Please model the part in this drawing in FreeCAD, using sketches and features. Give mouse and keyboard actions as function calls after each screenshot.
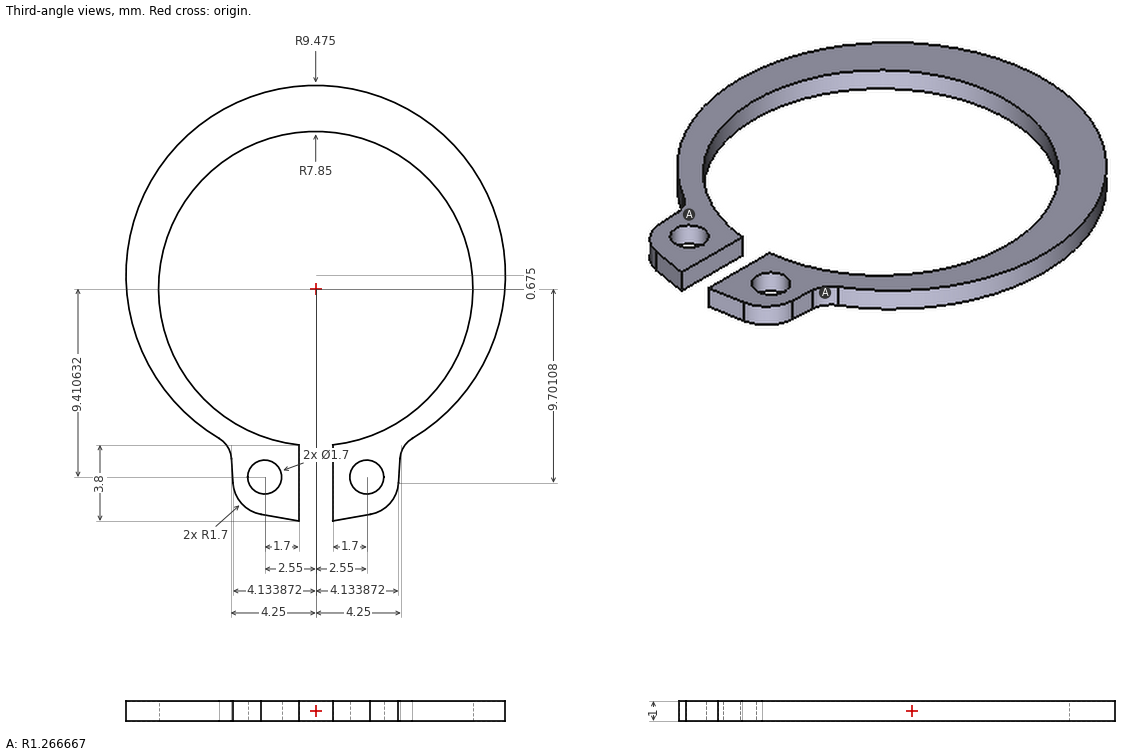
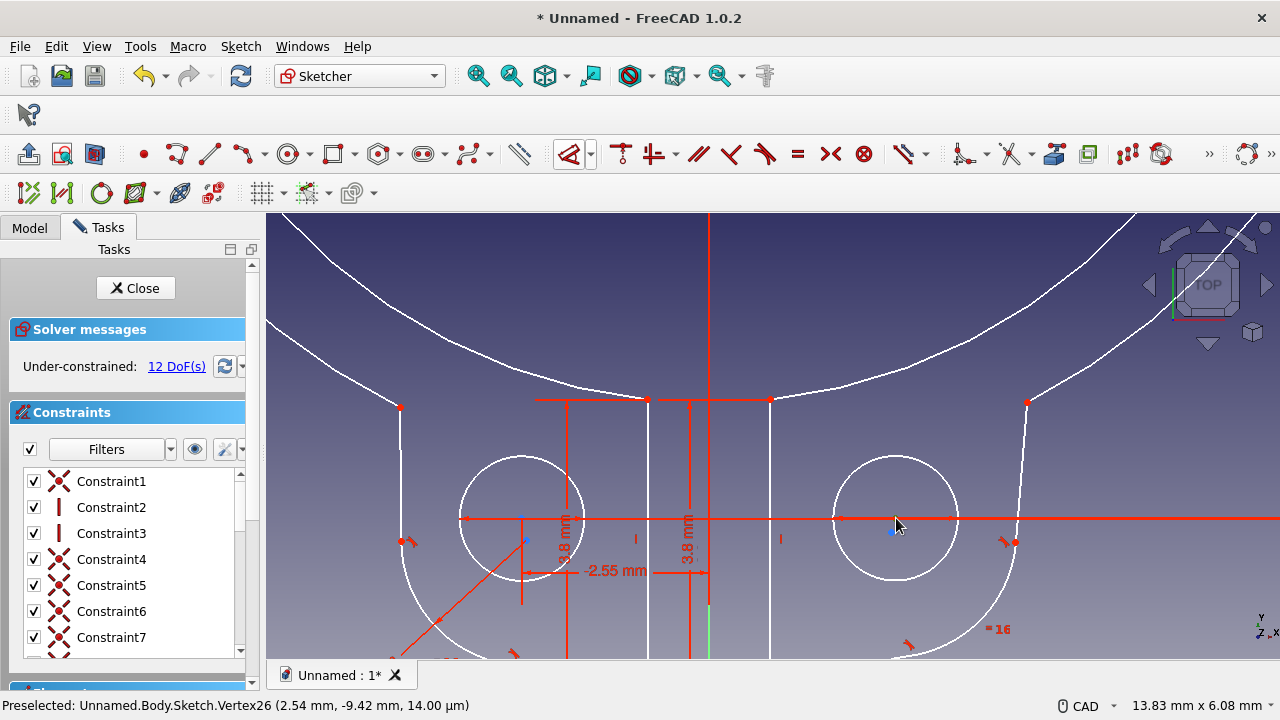
key(l)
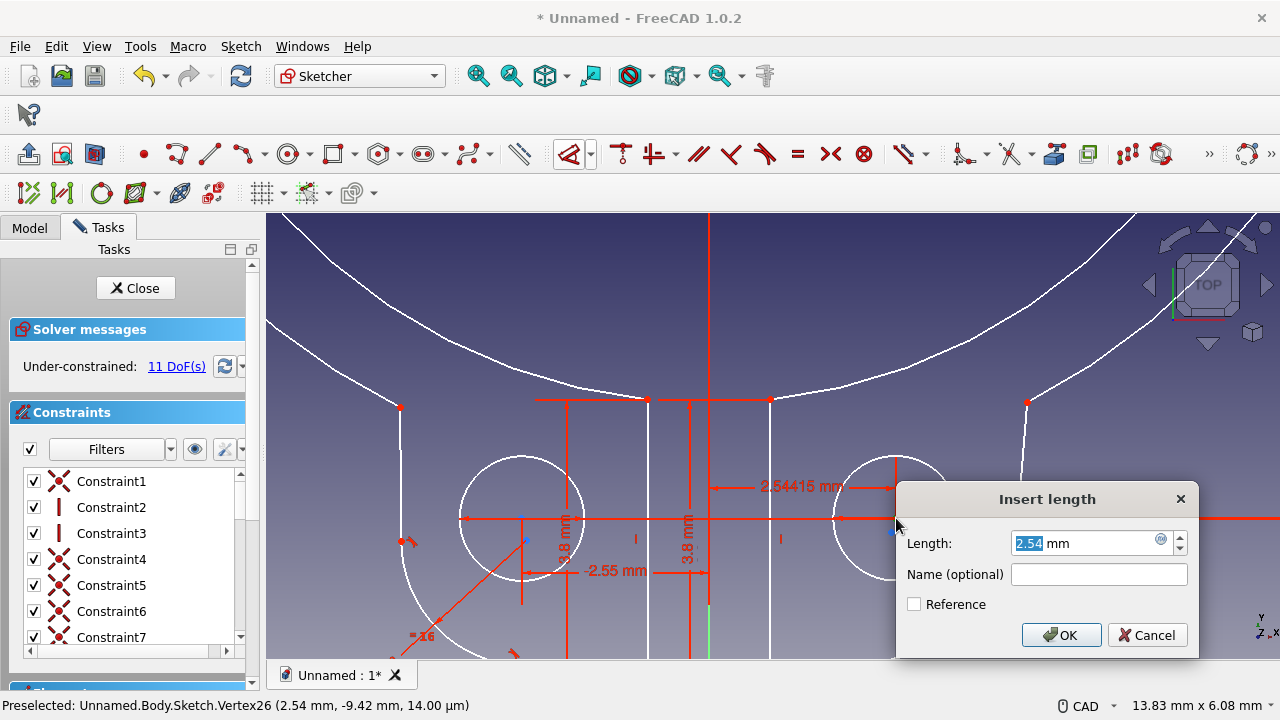
text(2.55)
key(Return)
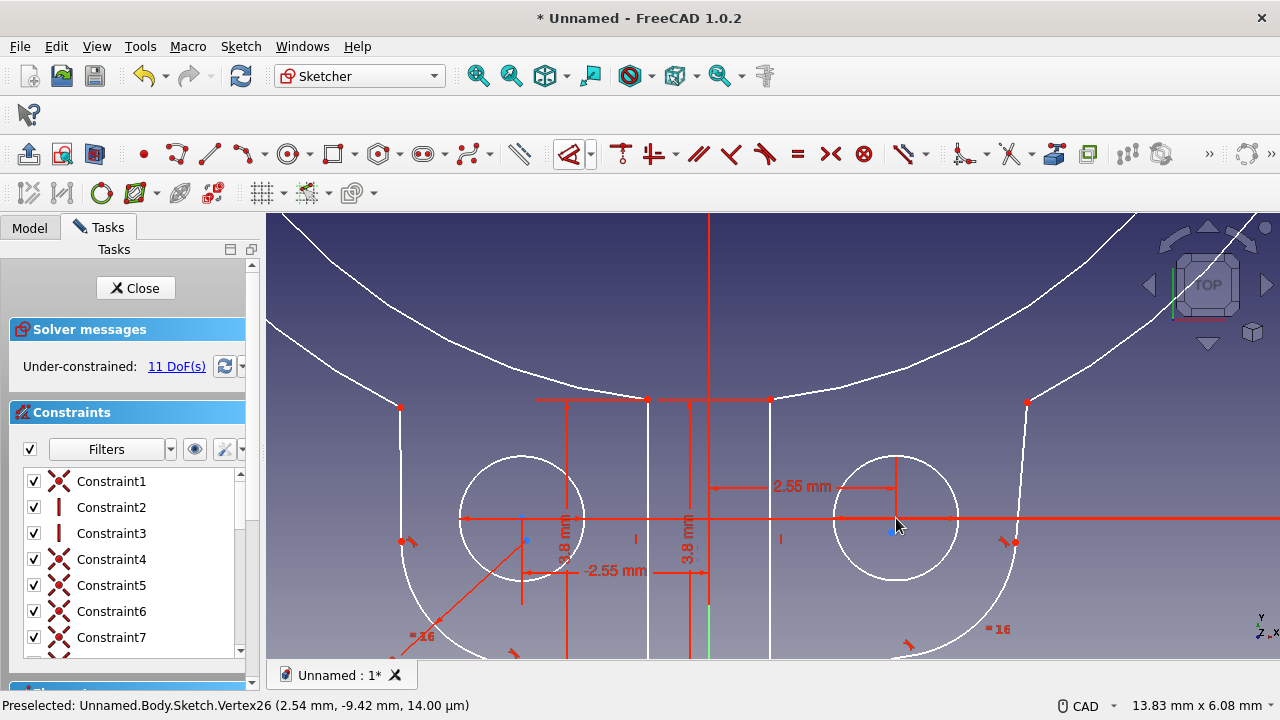
scroll(704, 546, down, 9)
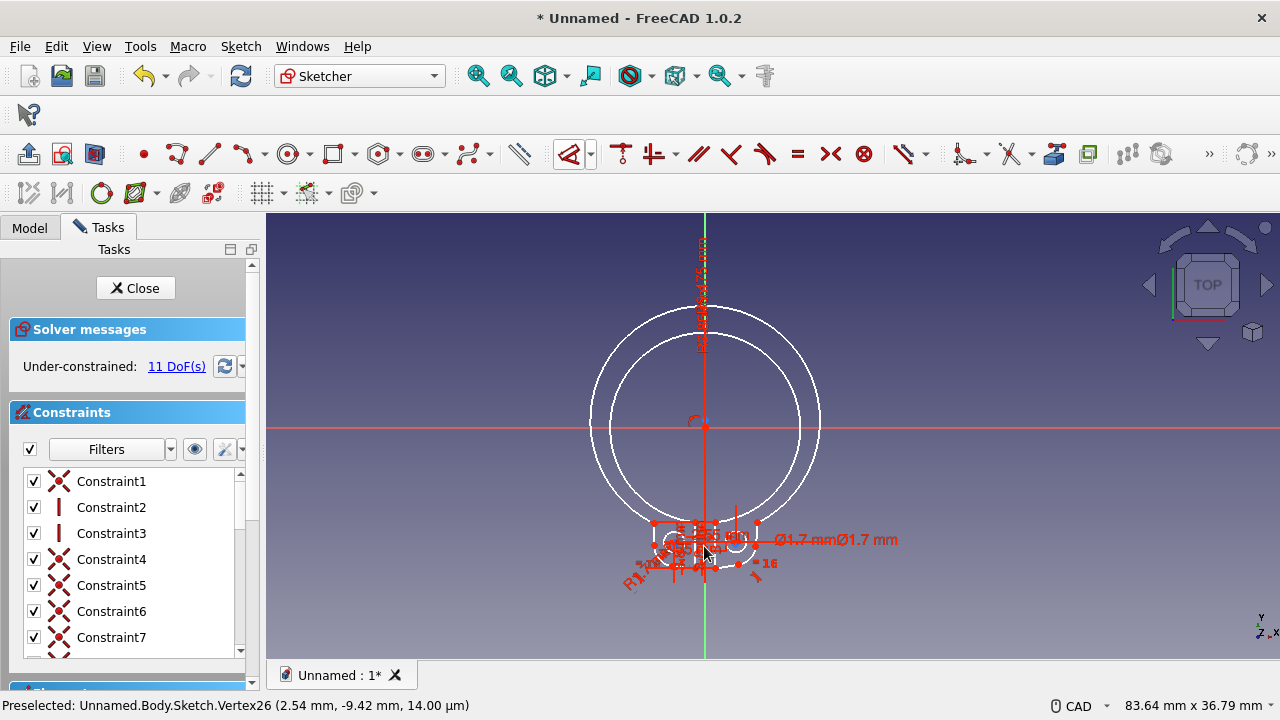
scroll(695, 522, up, 4)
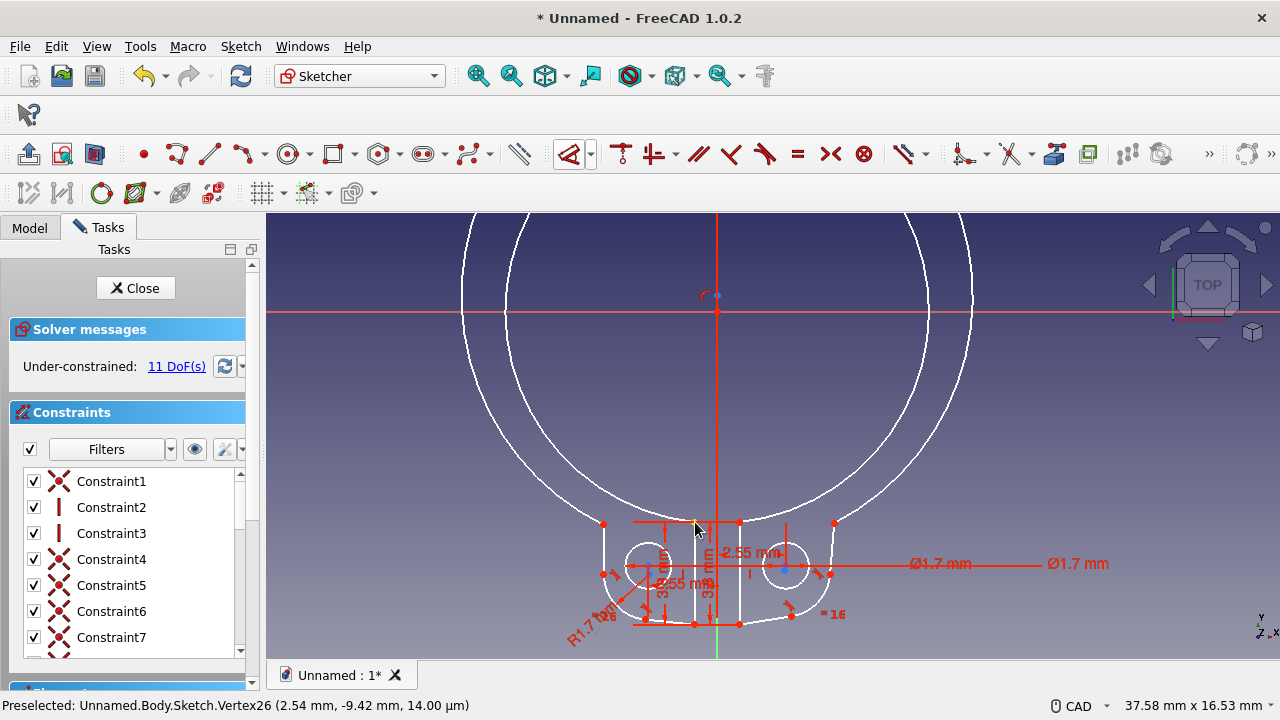
click(695, 522)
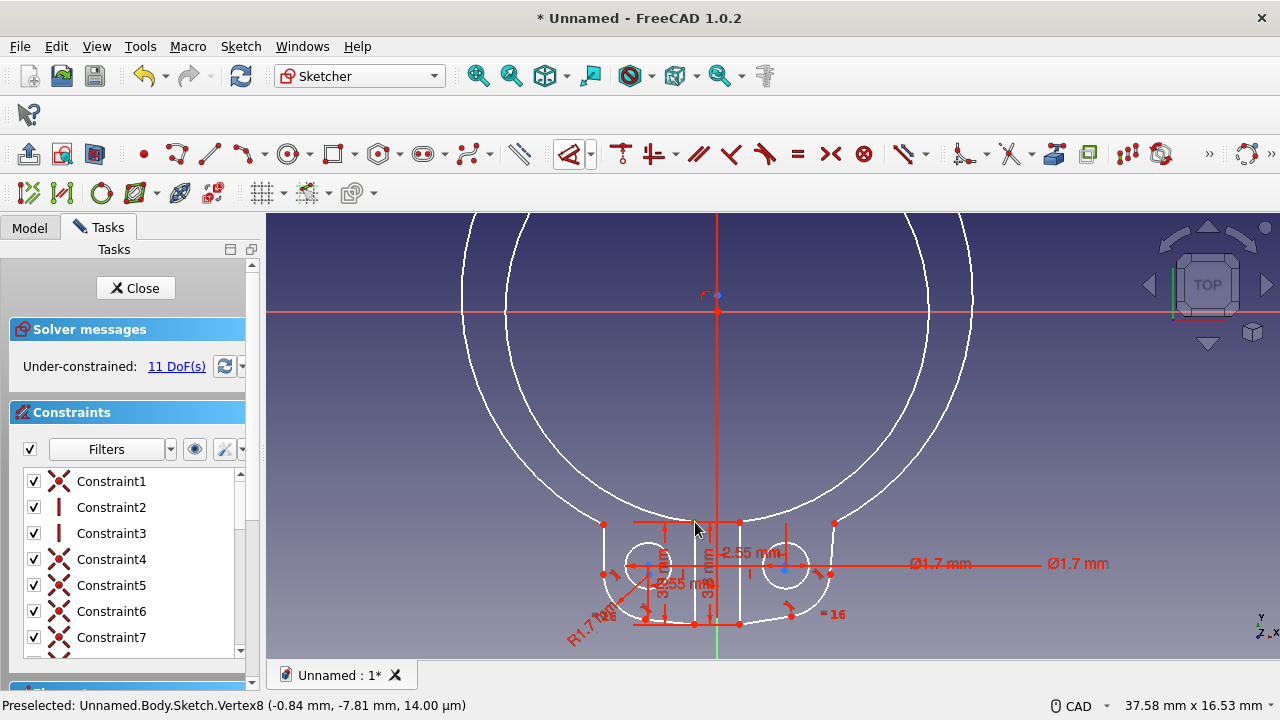
scroll(648, 566, up, 2)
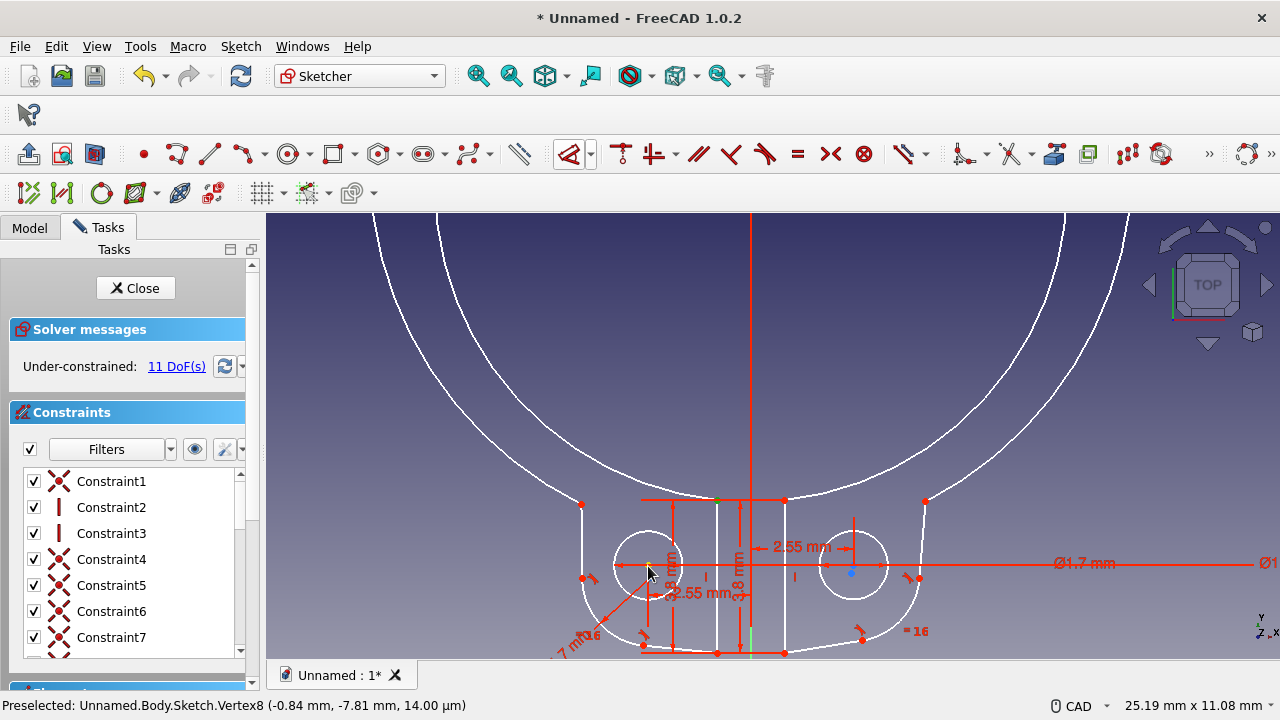
click(648, 565)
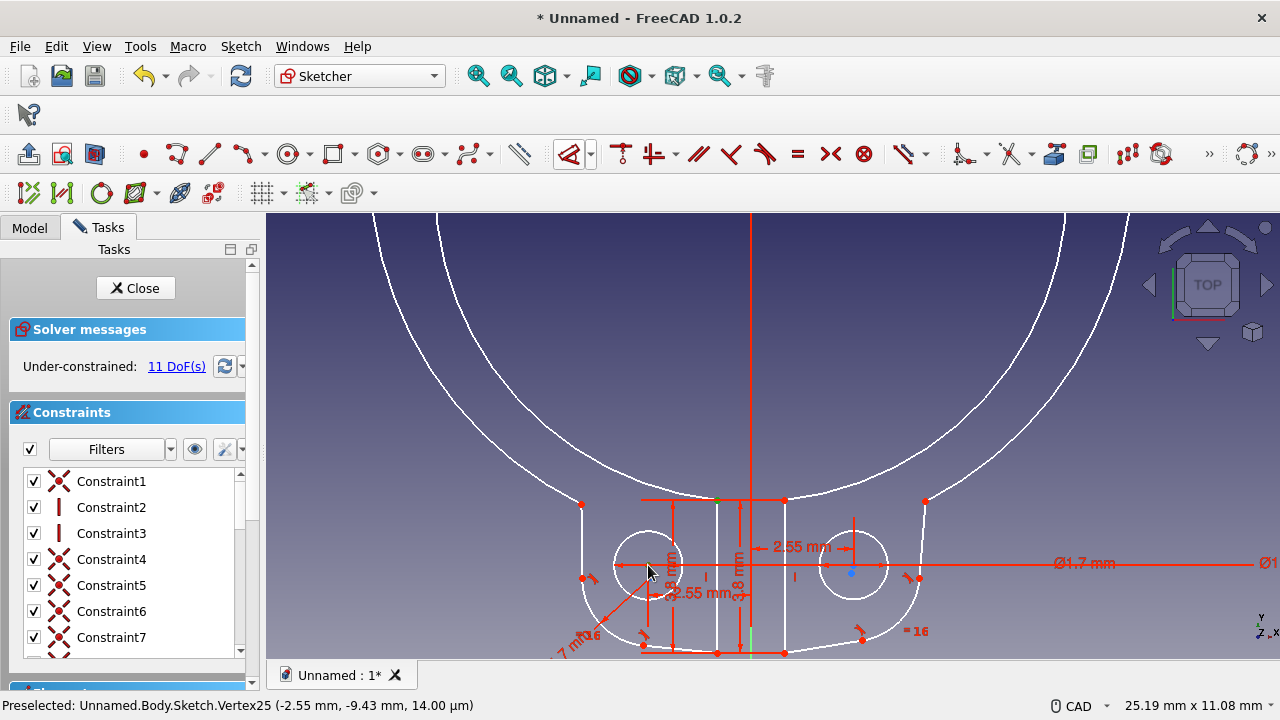
key(l)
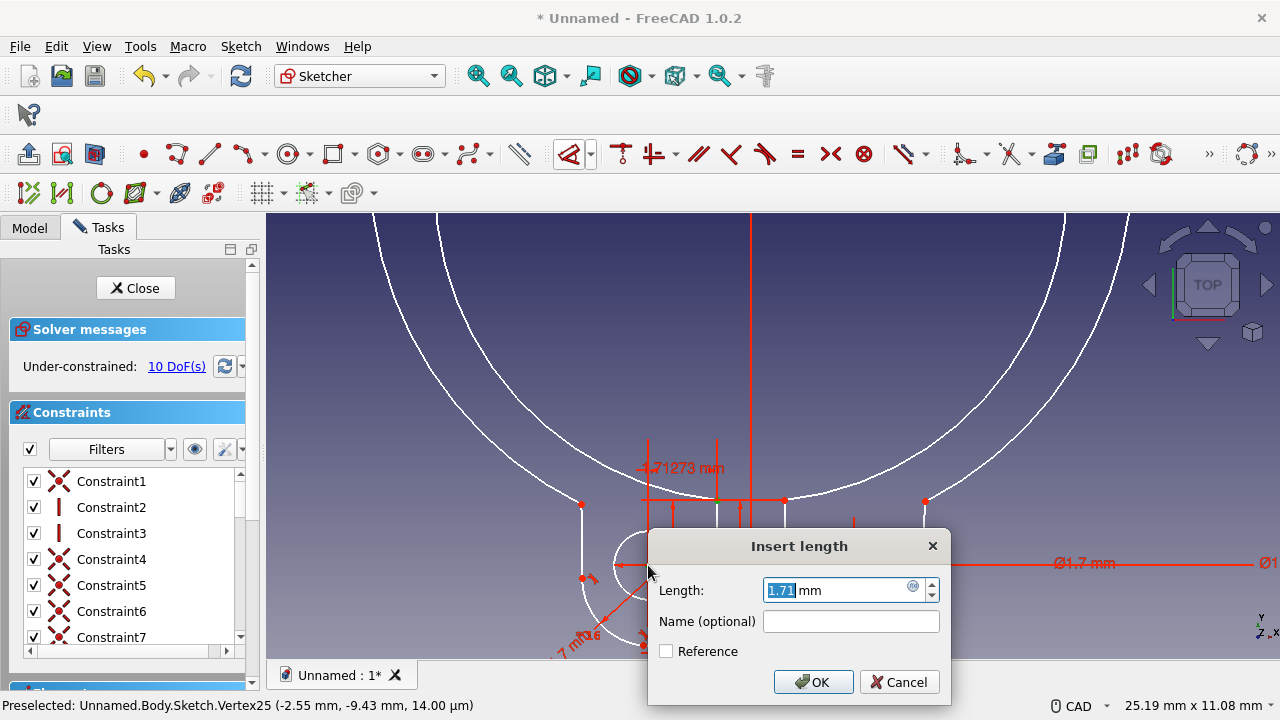
text(1.7)
key(Return)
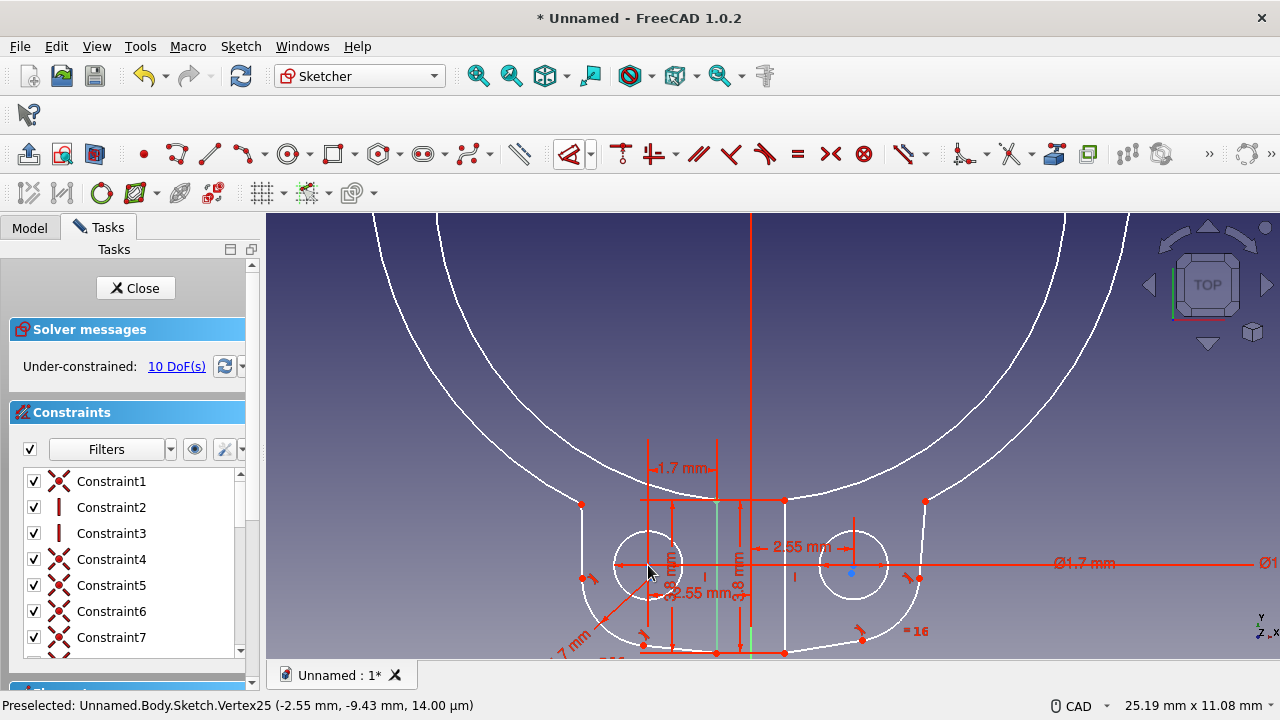
click(785, 500)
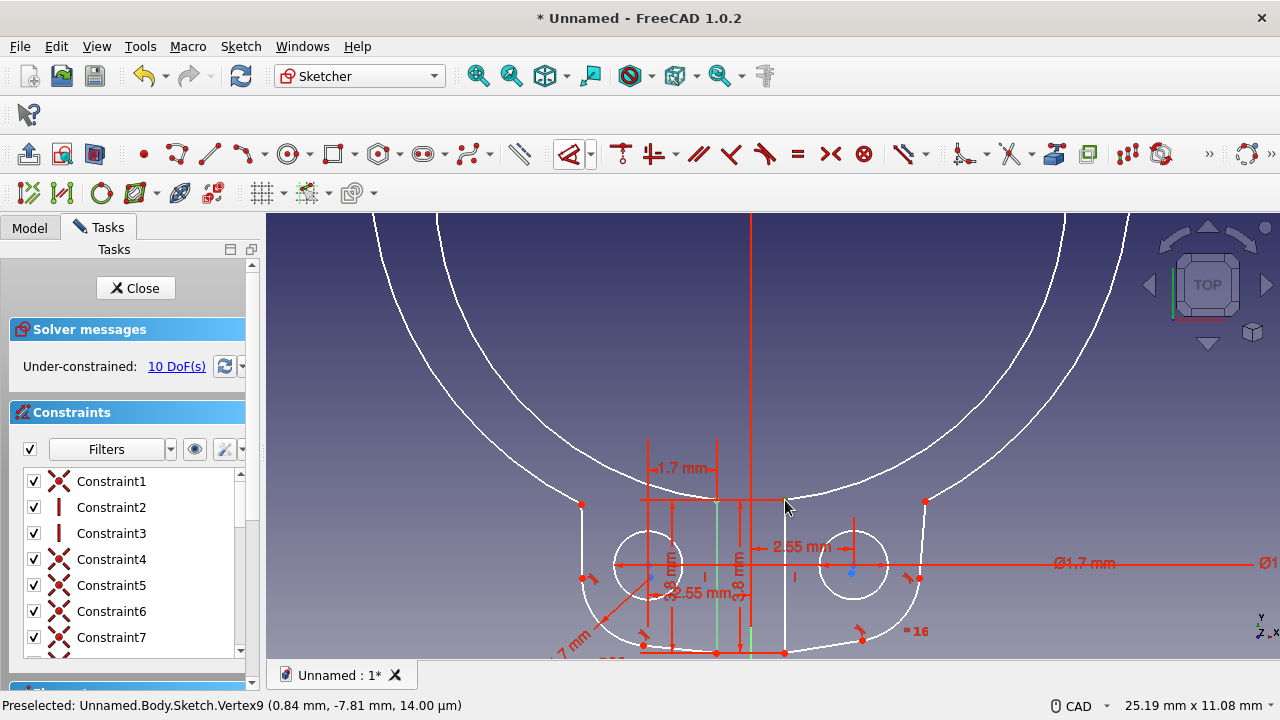
scroll(854, 565, up, 2)